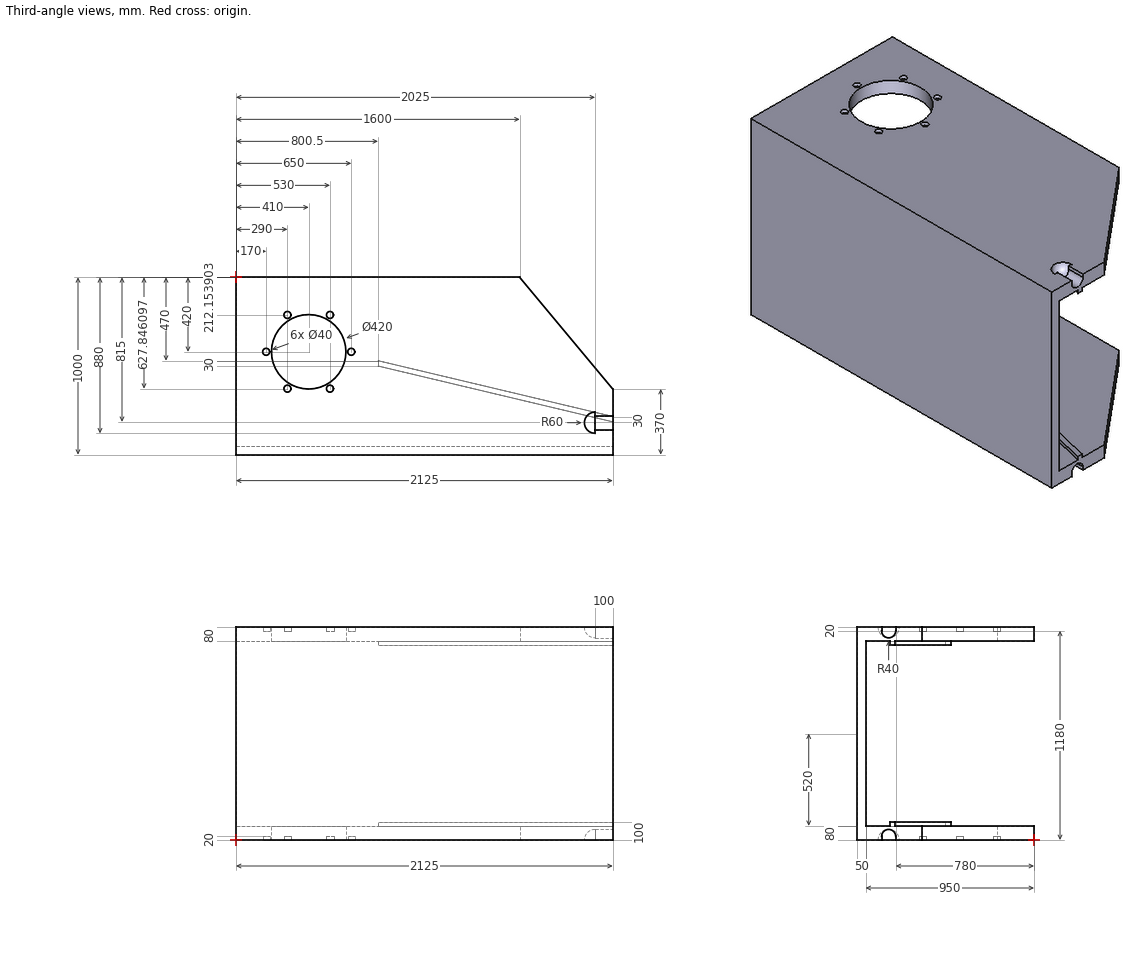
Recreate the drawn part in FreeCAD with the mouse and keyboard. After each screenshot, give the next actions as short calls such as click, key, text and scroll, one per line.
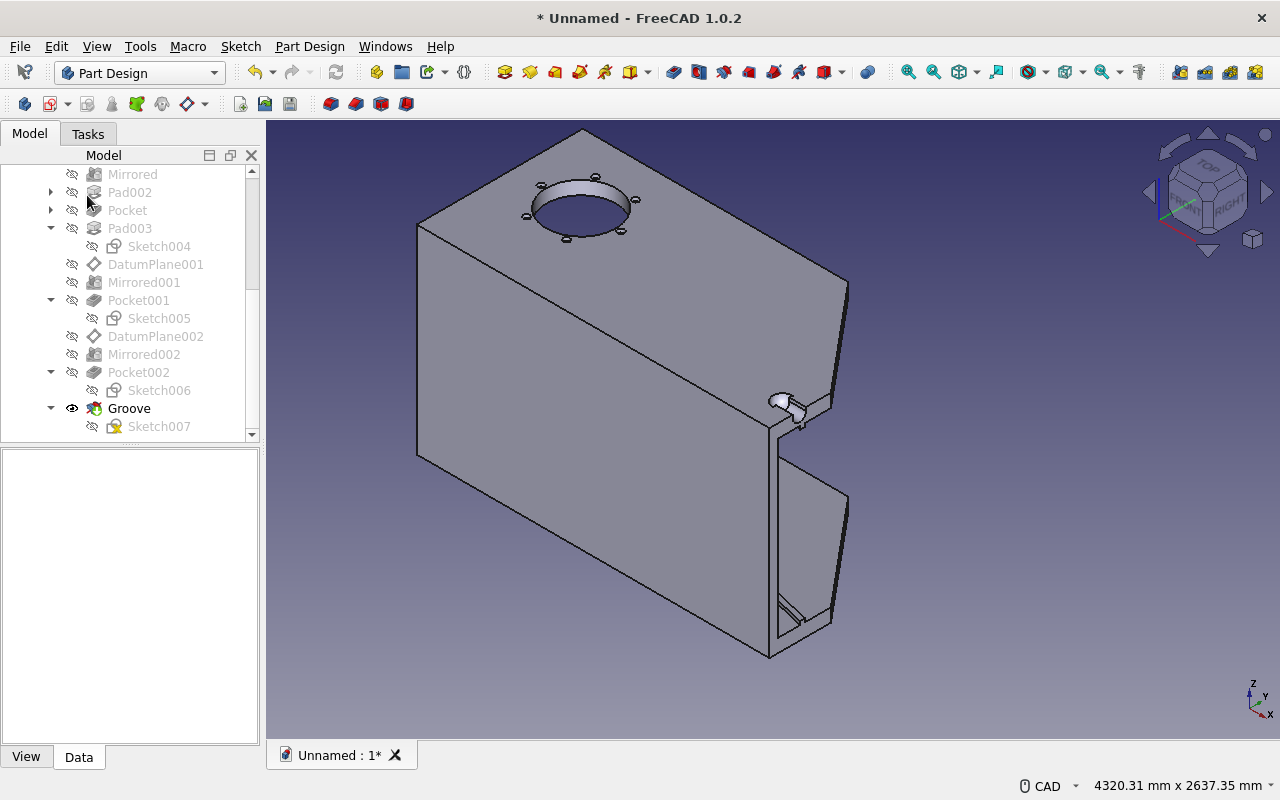
scroll(141, 296, down, 3)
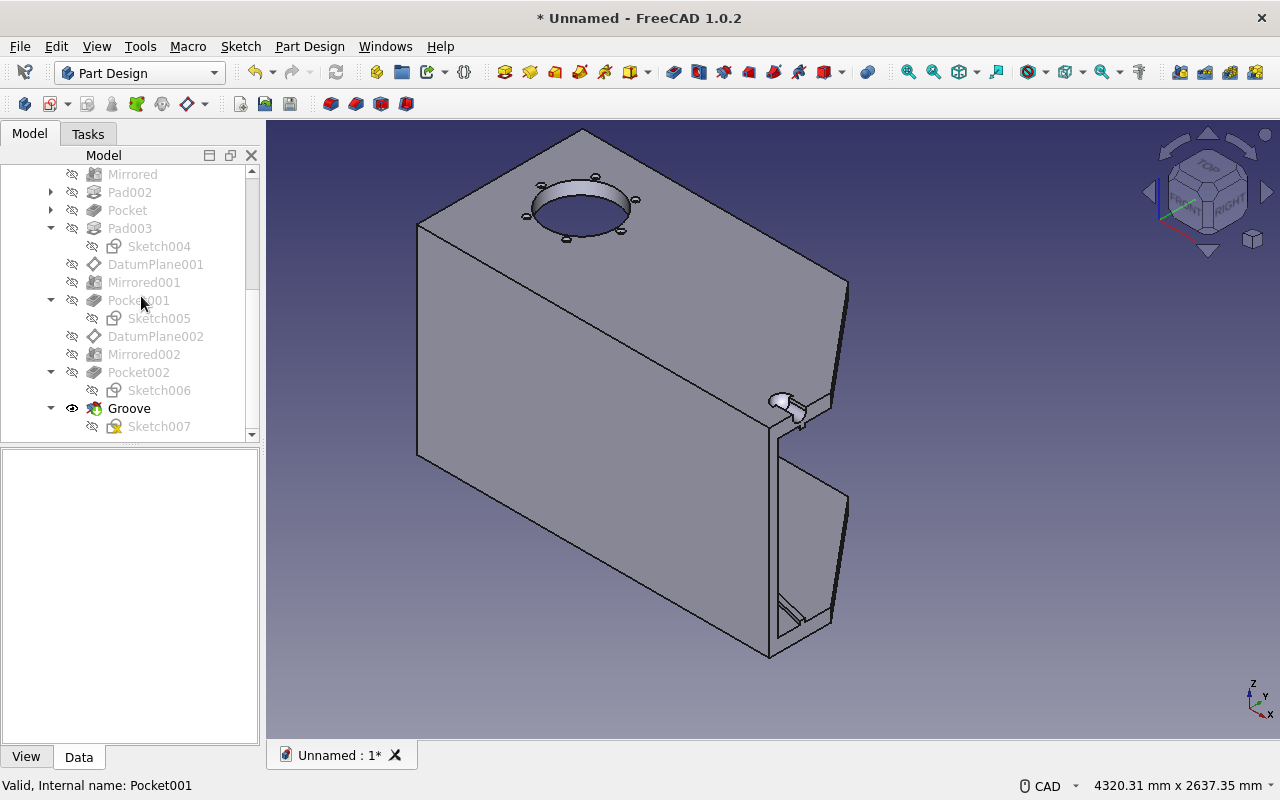
scroll(141, 296, up, 15)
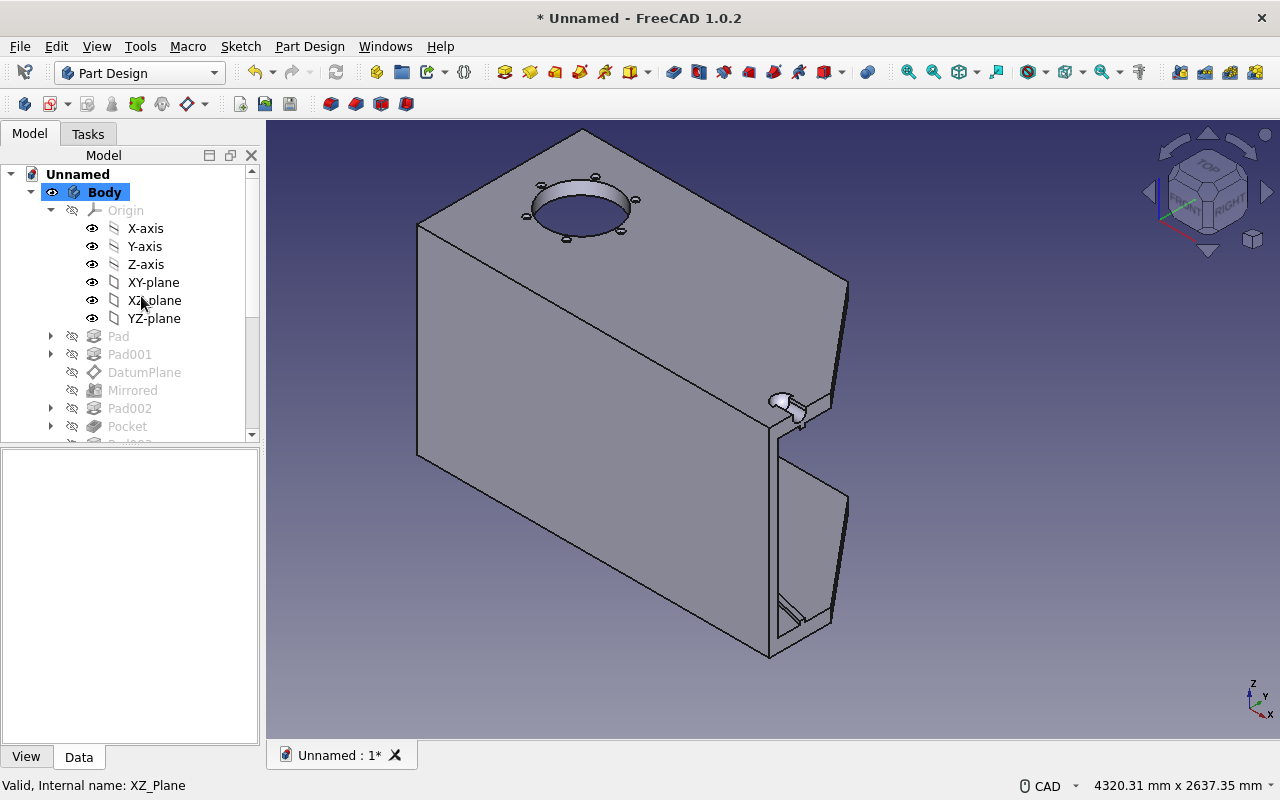
click(137, 282)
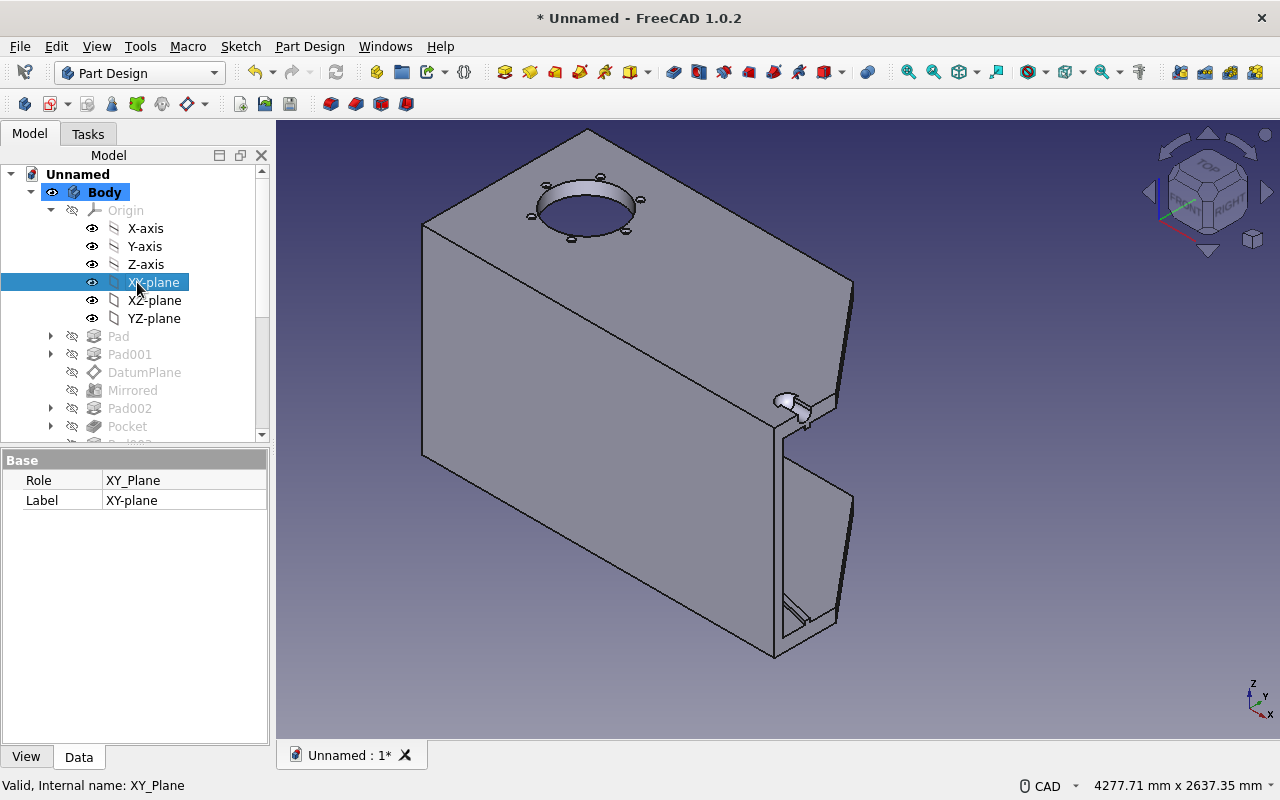
click(186, 104)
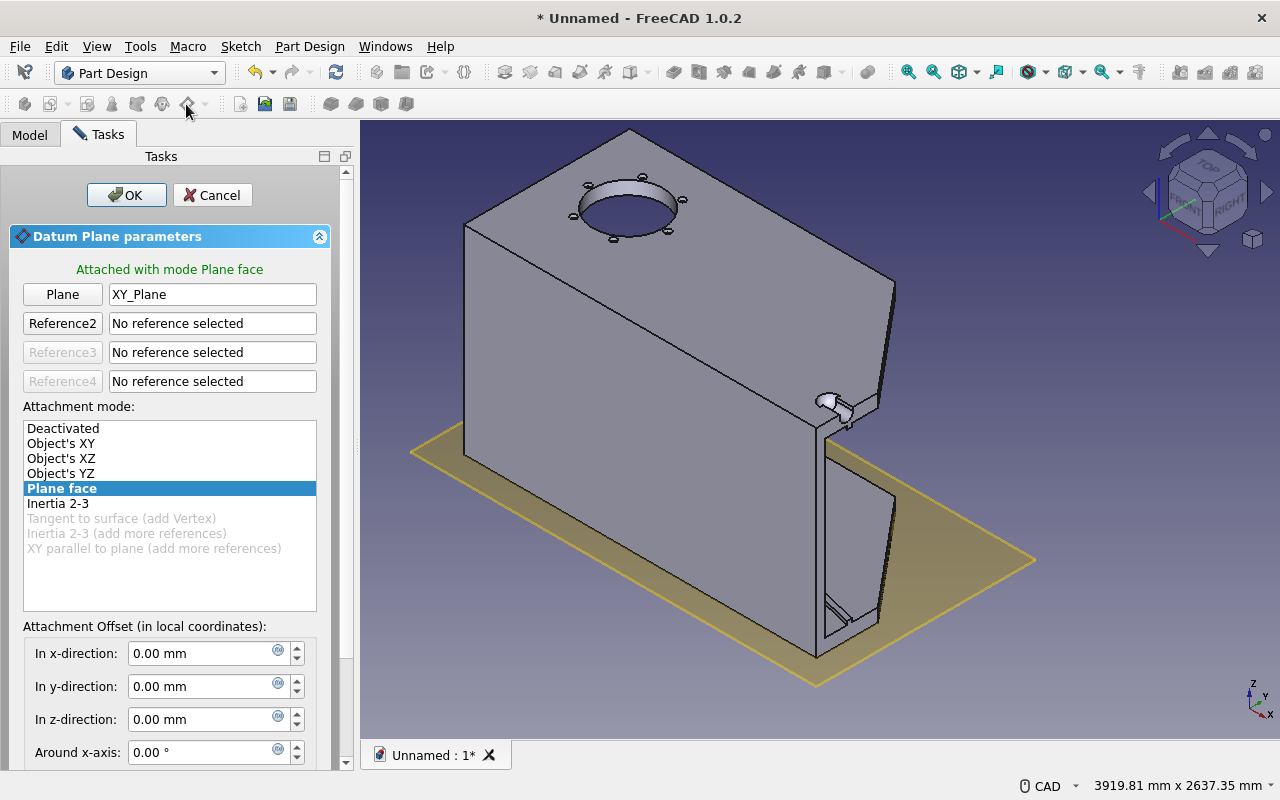
triple_click(210, 720)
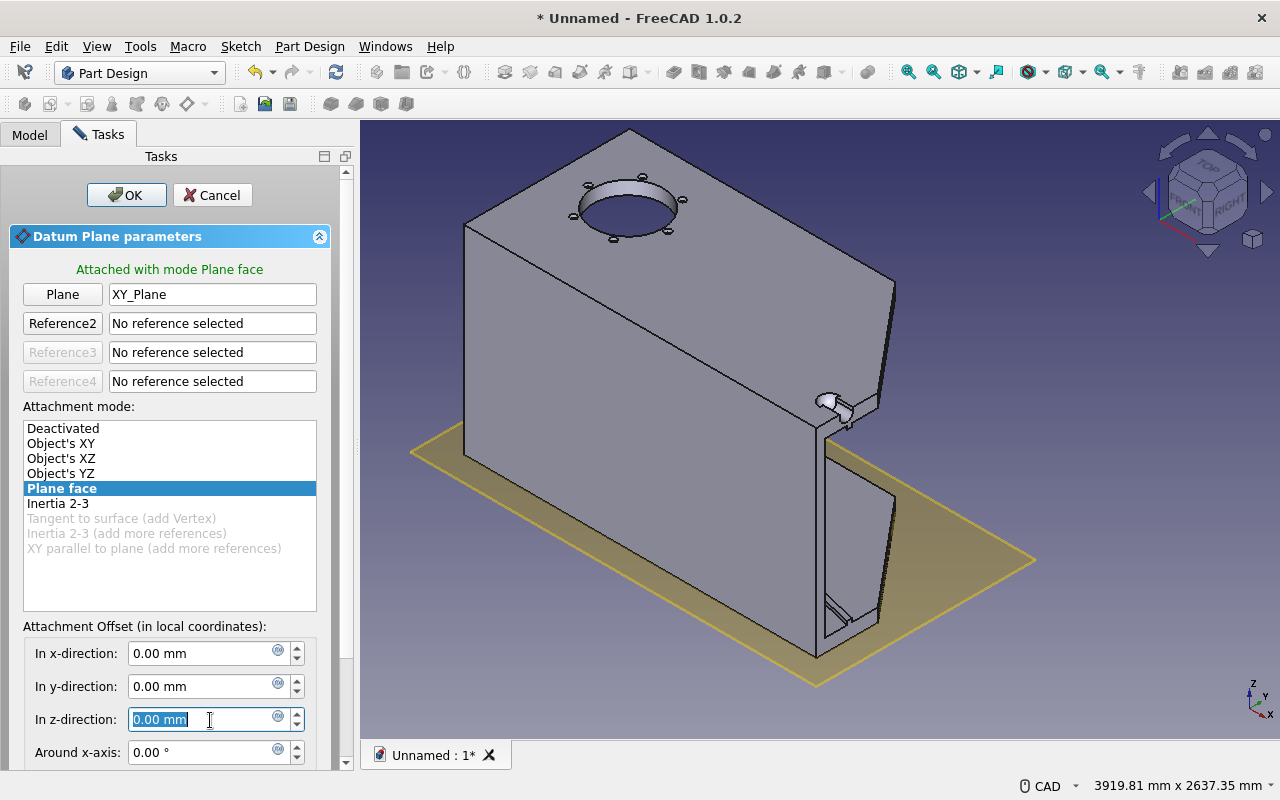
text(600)
key(Tab)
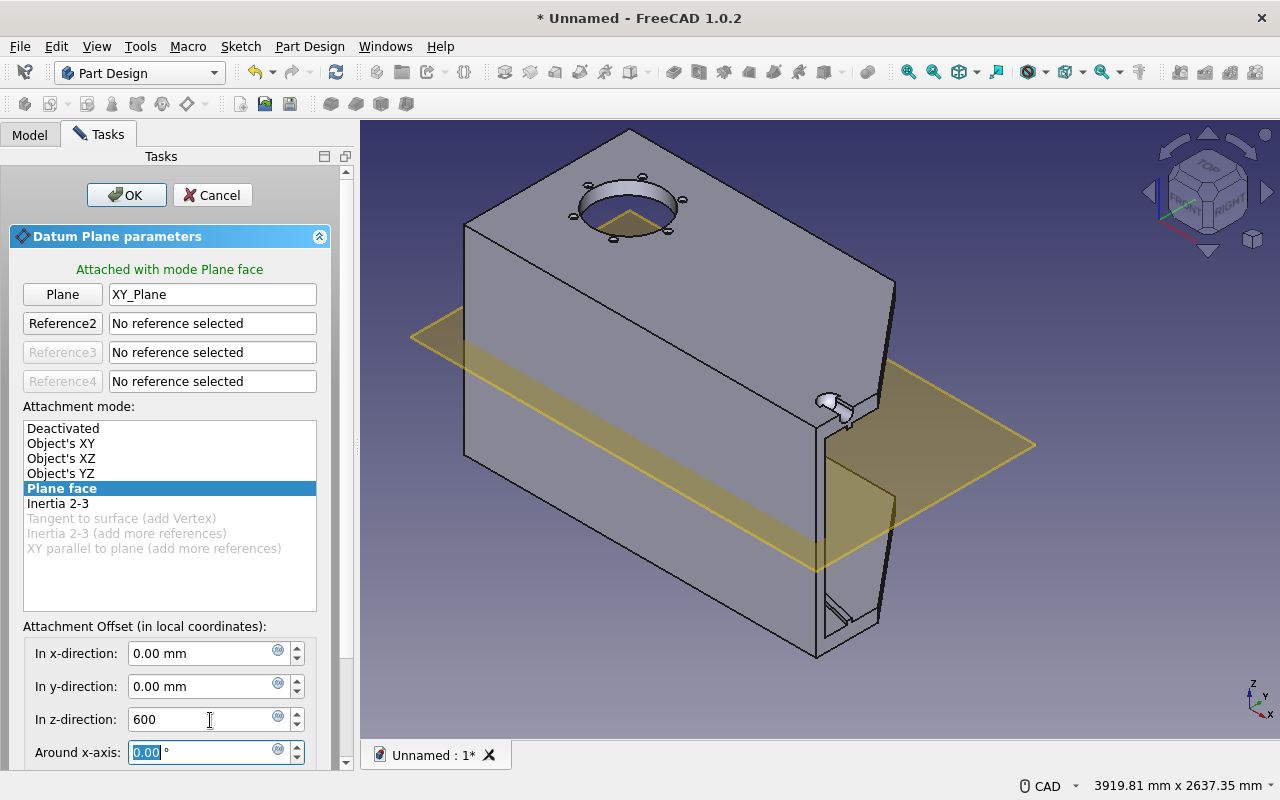
click(127, 195)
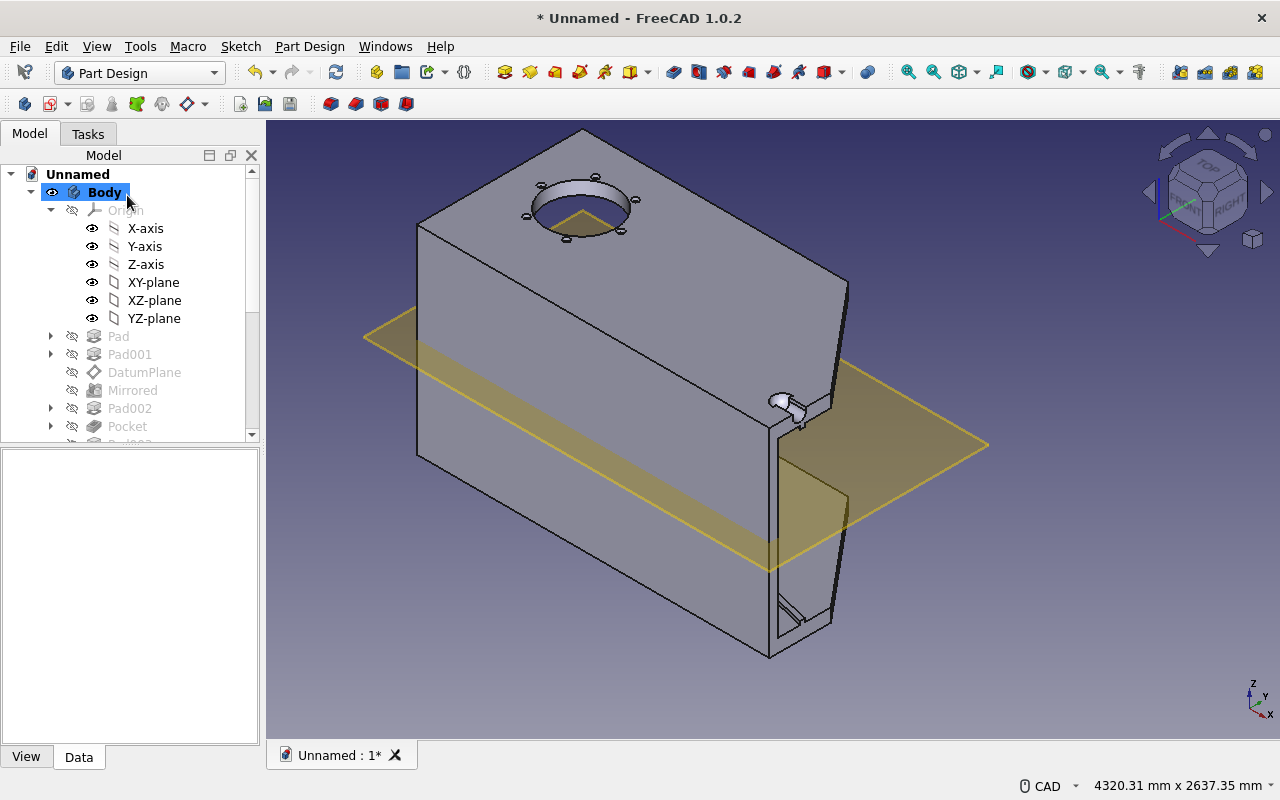
scroll(101, 296, down, 3)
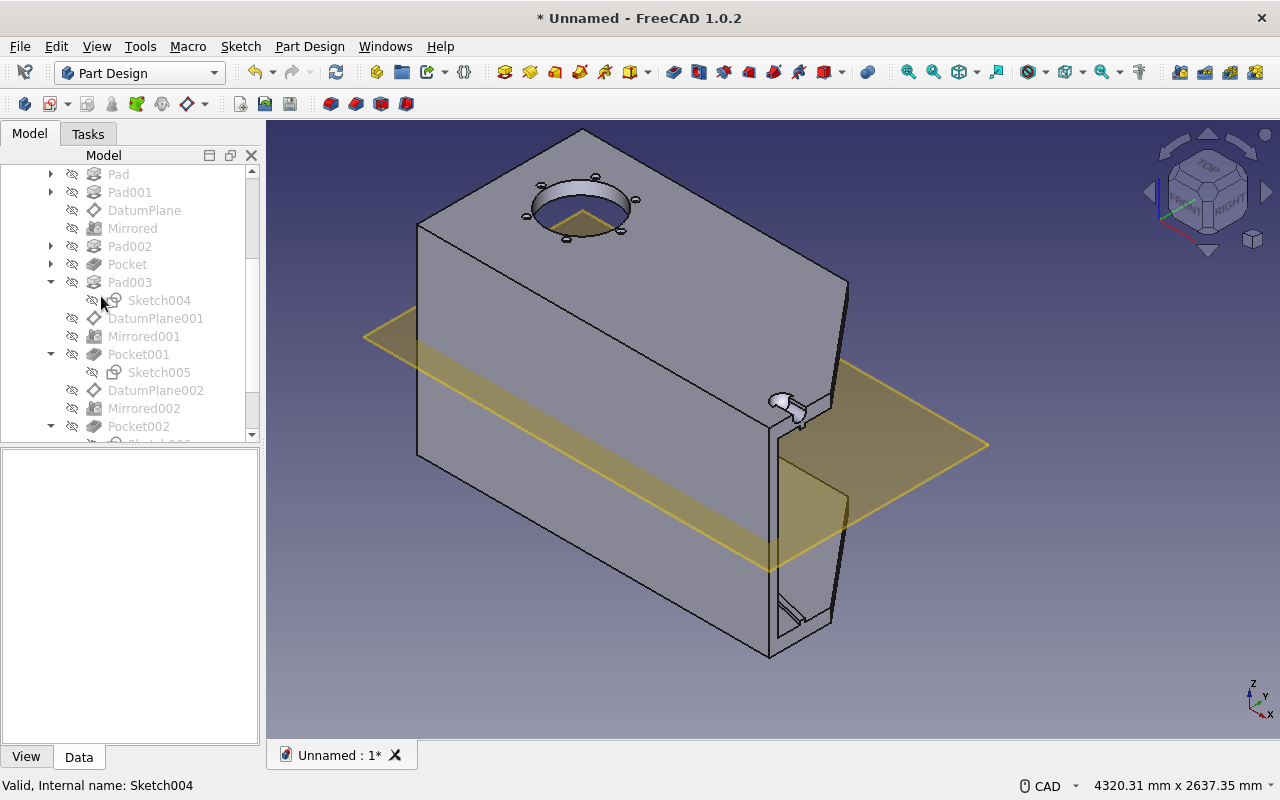
click(117, 426)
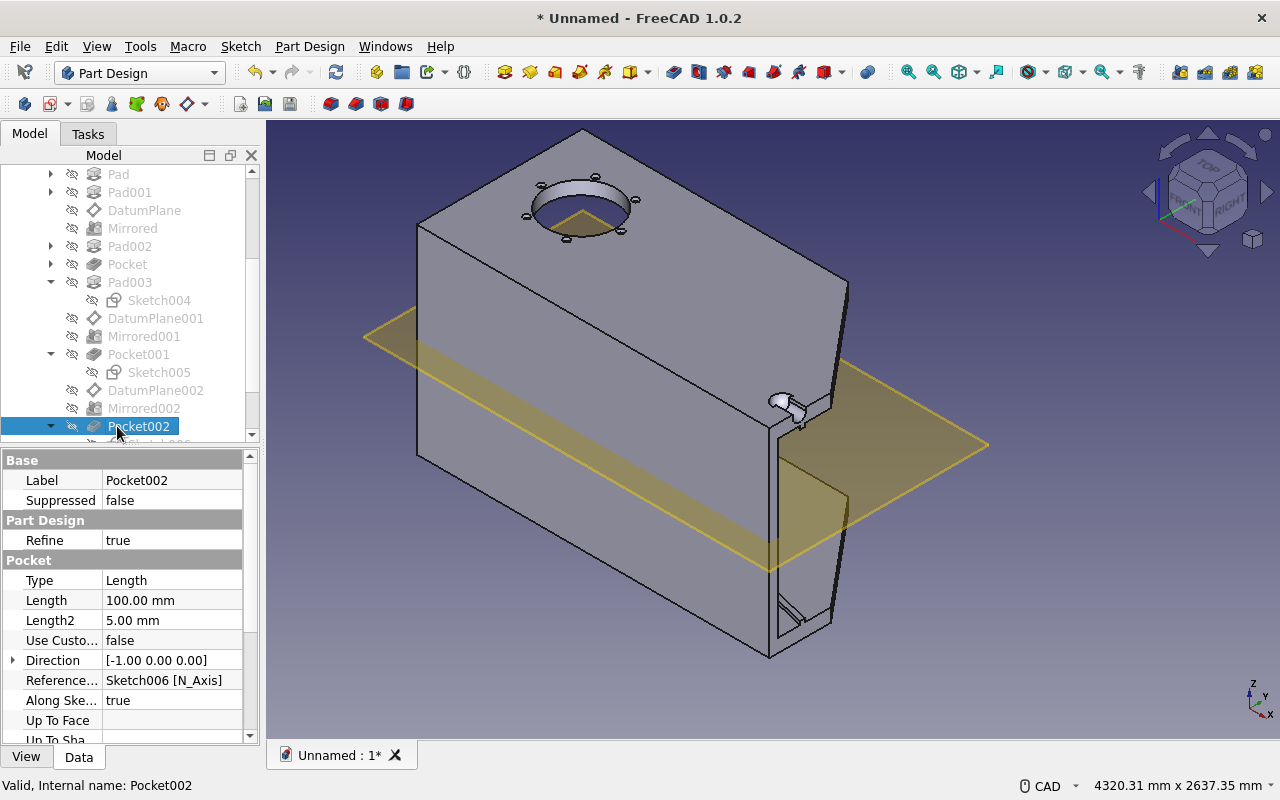
scroll(141, 296, down, 3)